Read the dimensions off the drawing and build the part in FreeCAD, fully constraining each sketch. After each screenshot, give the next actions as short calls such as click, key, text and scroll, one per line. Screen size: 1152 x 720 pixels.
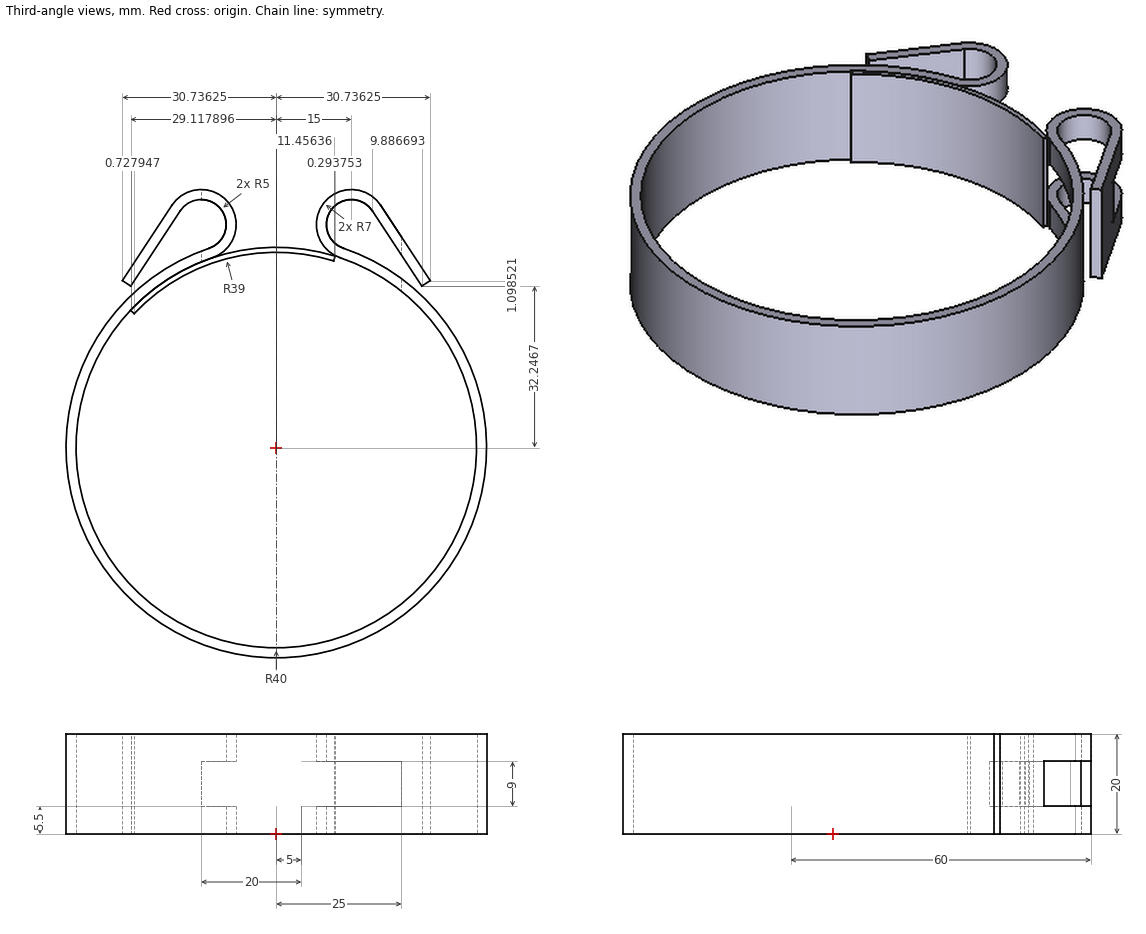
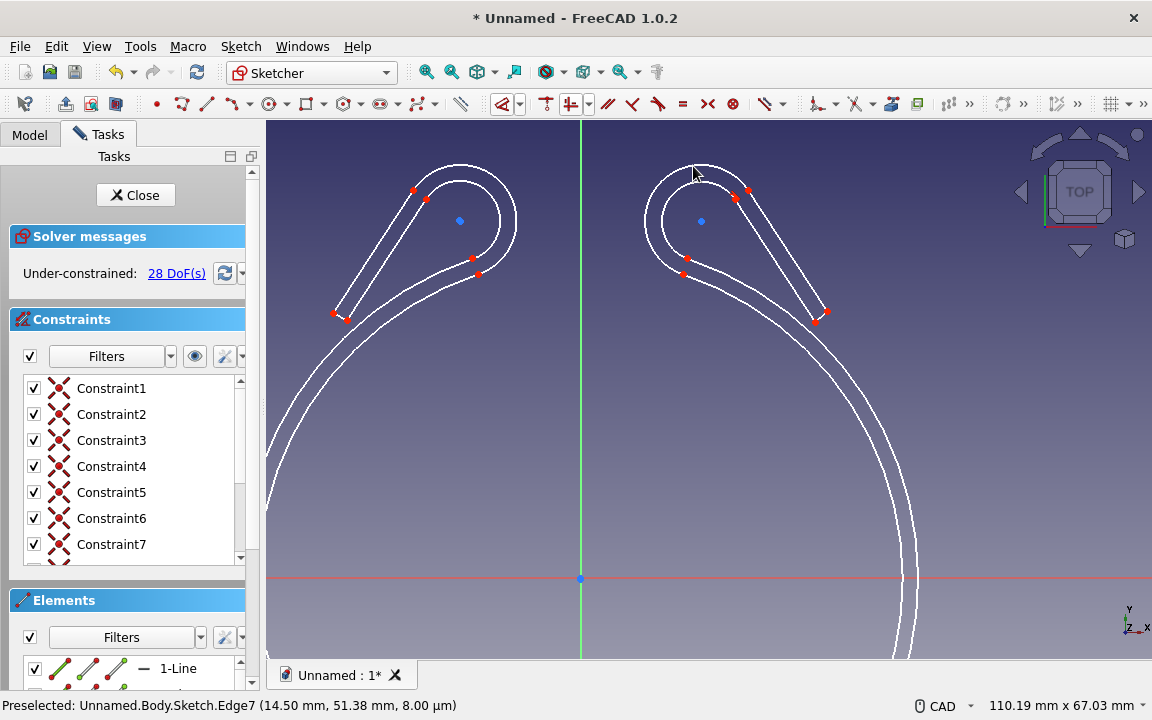
click(389, 227)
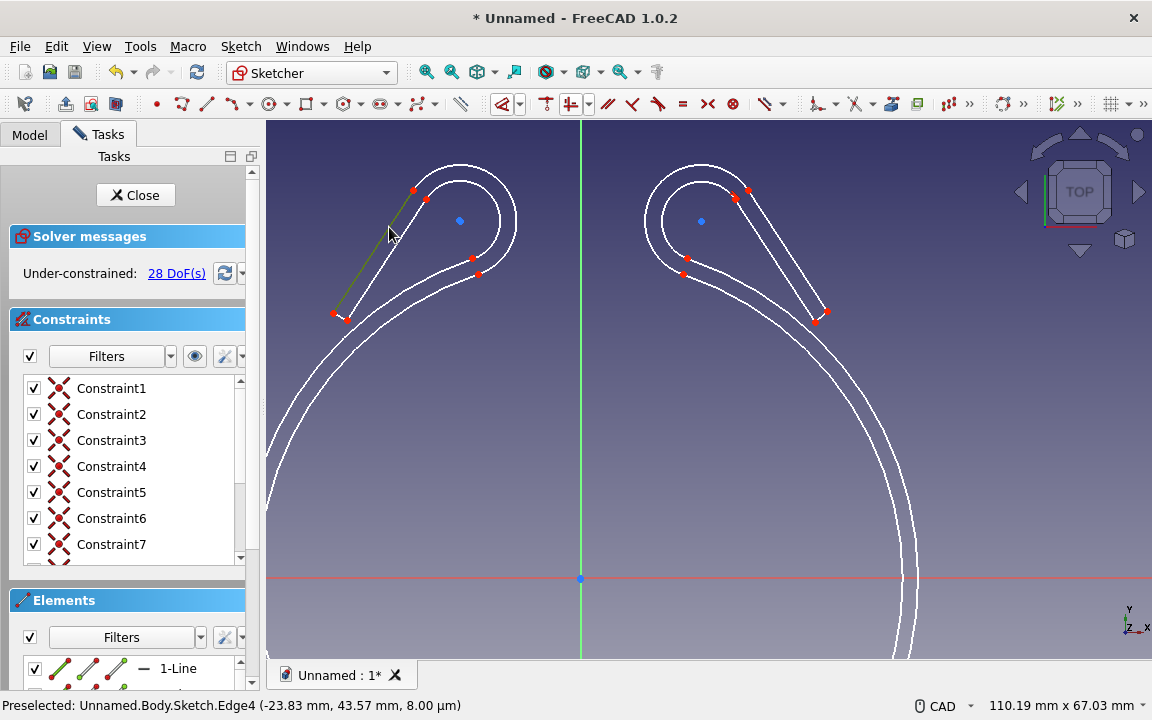
click(516, 227)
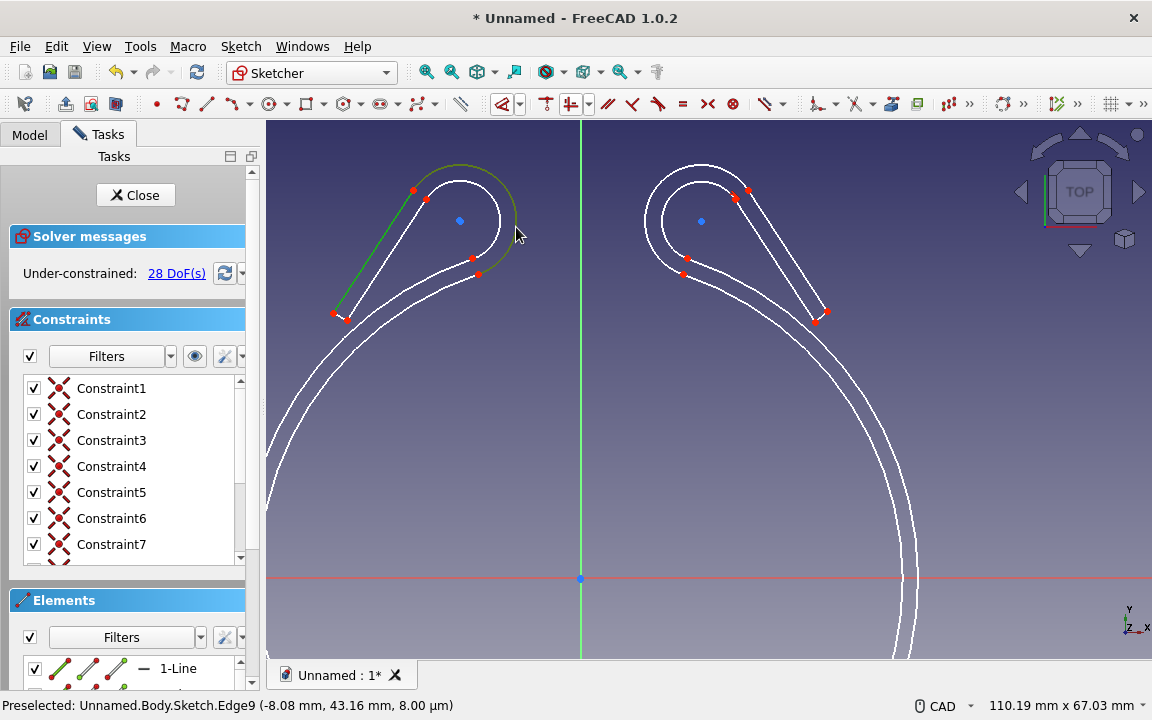
key(t)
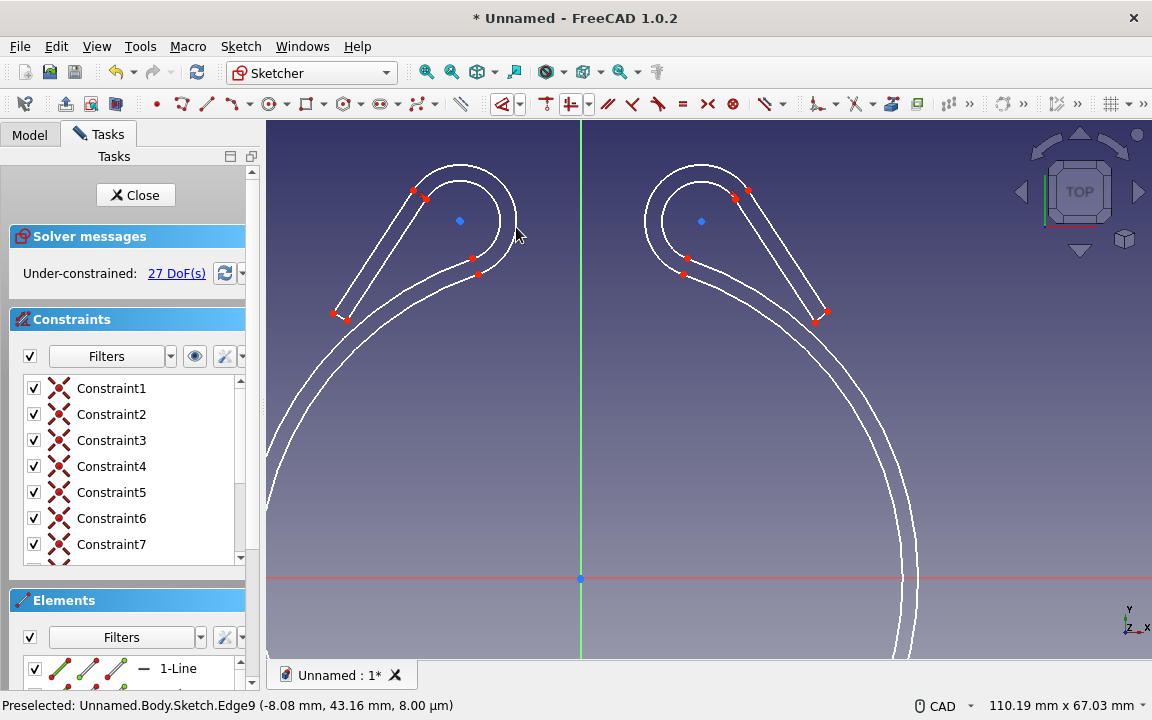
click(371, 284)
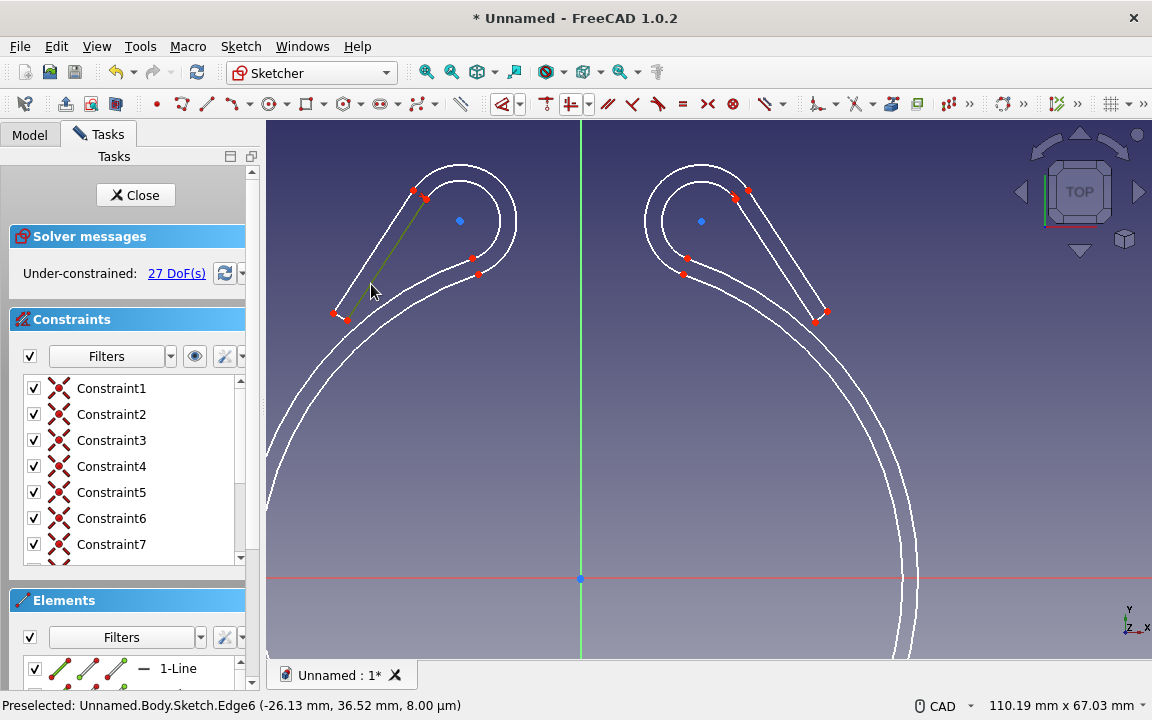
click(500, 225)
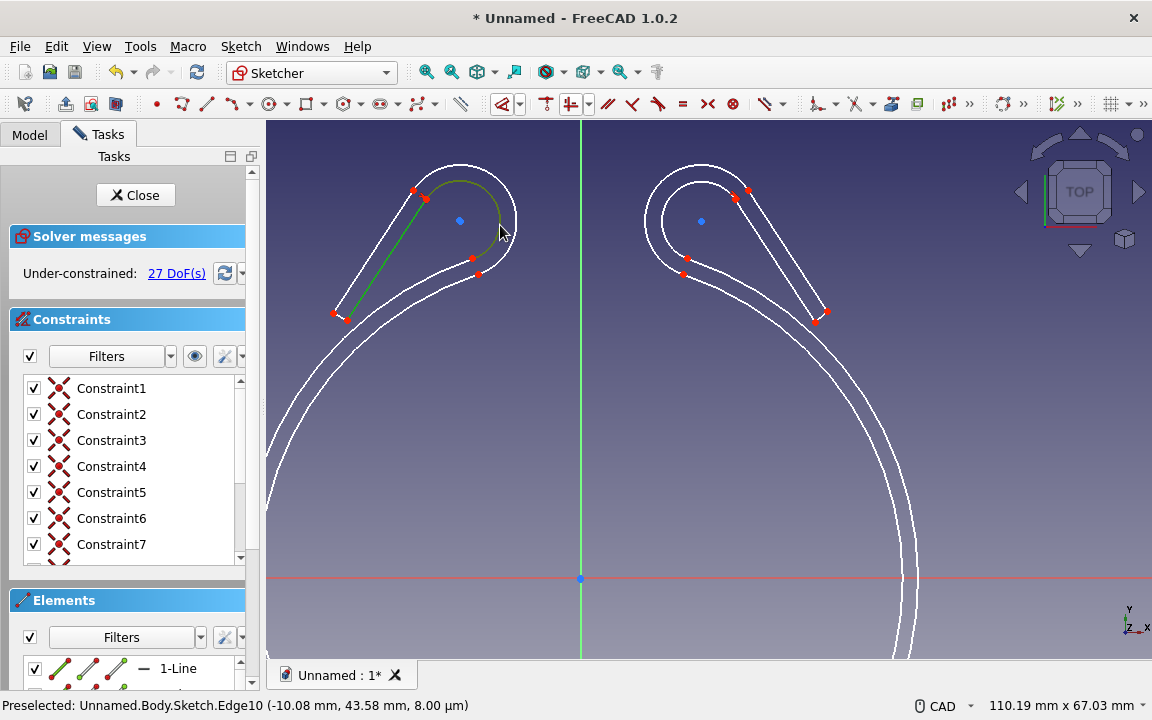
click(658, 104)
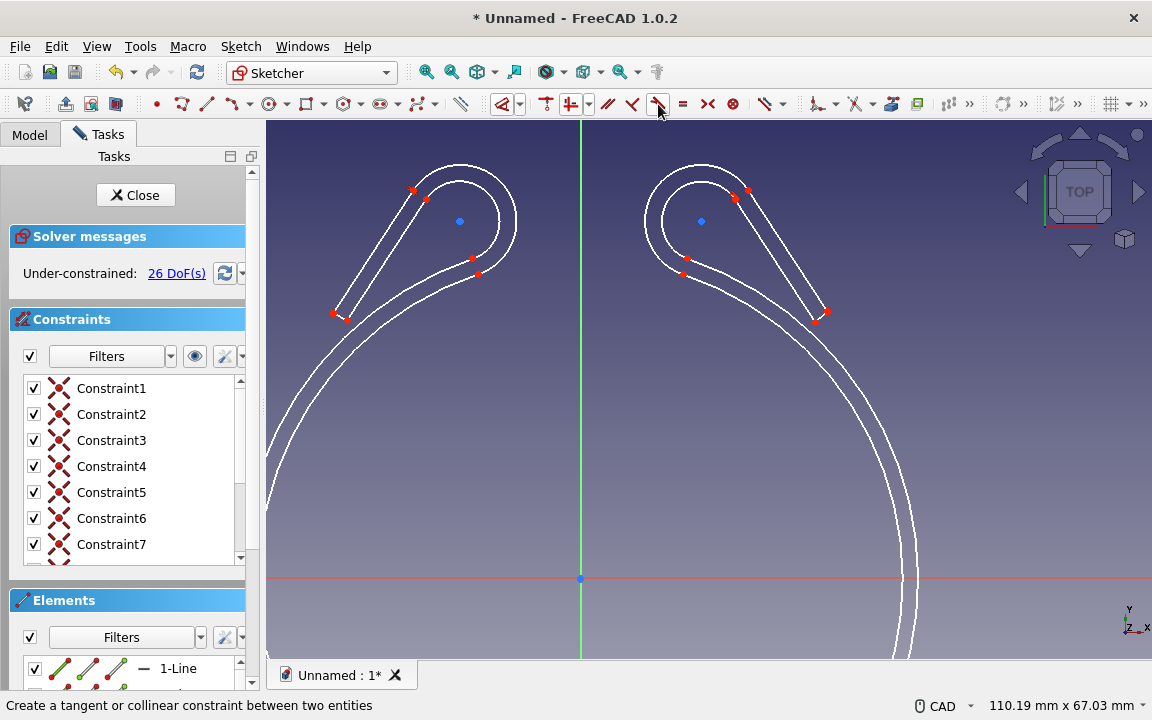
click(693, 166)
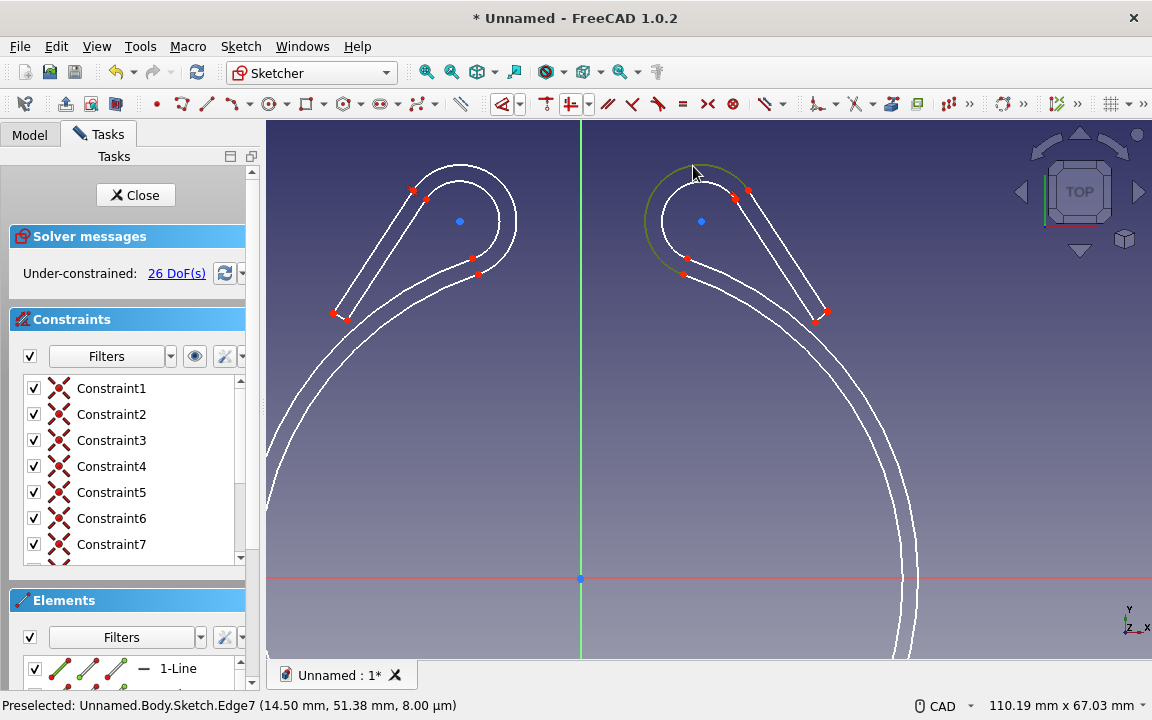
click(900, 541)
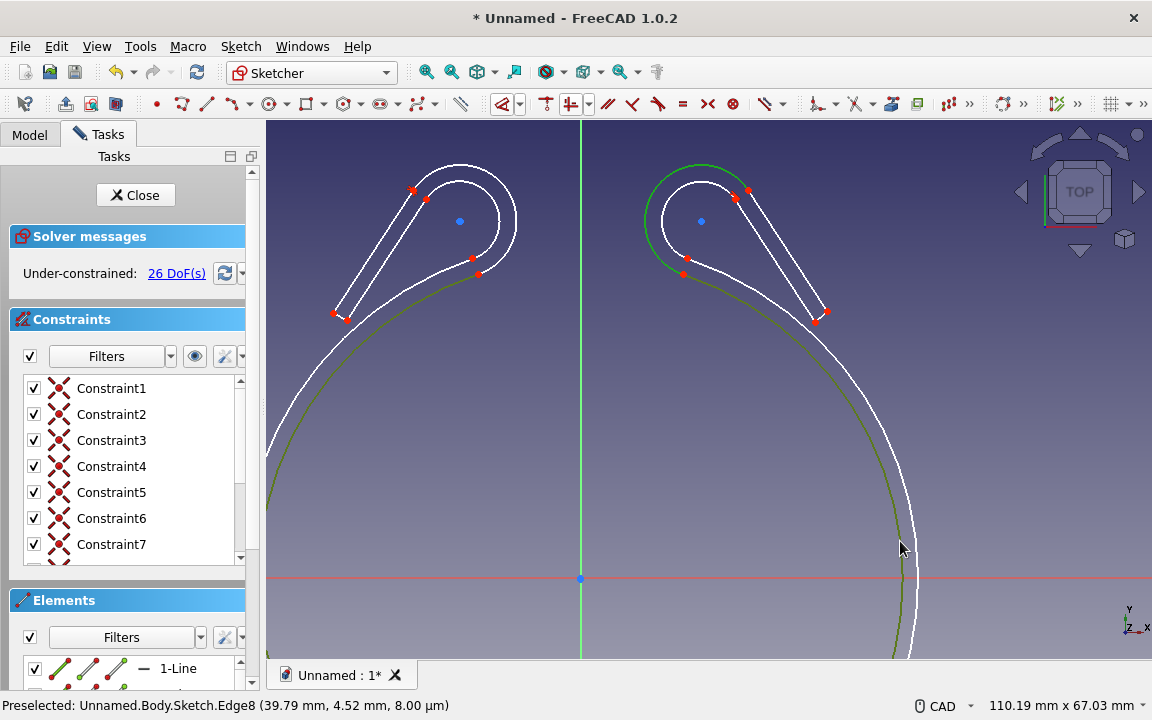
key(t)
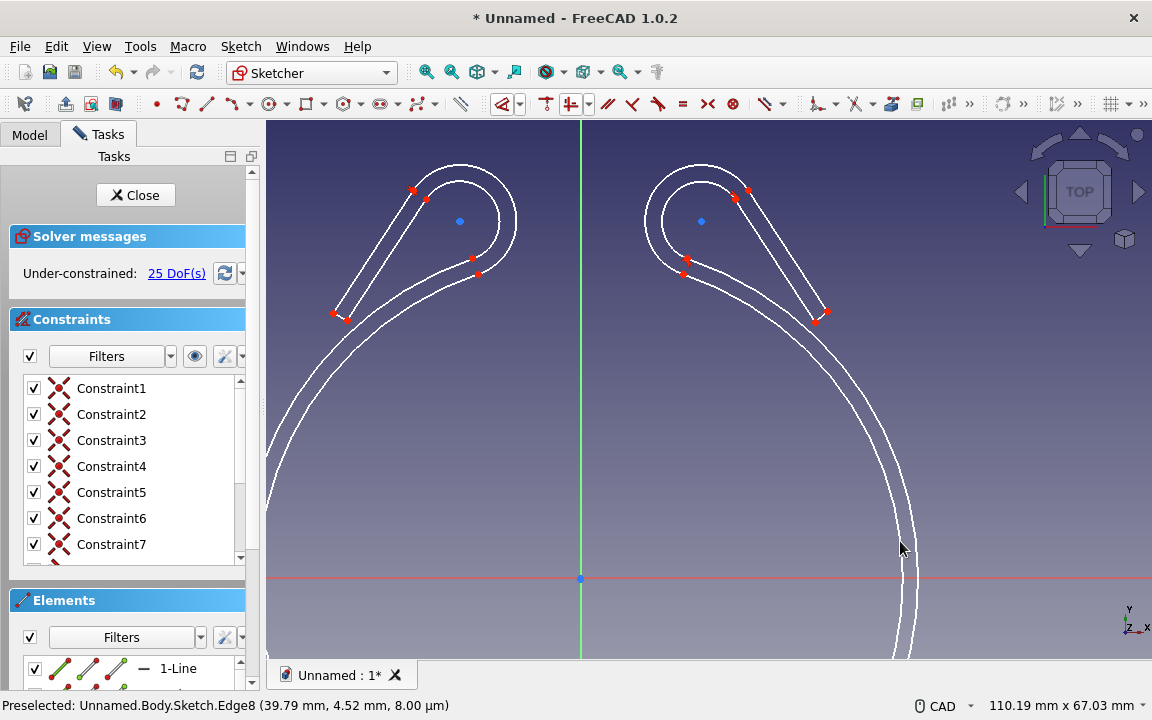
click(901, 542)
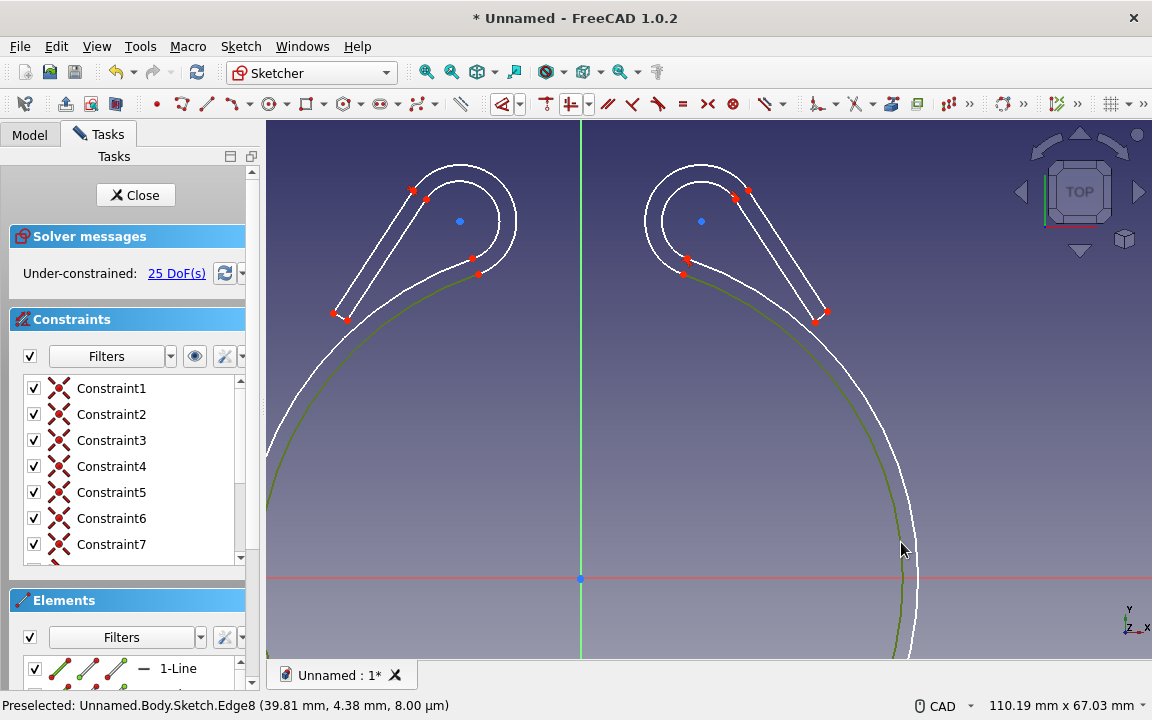
click(516, 227)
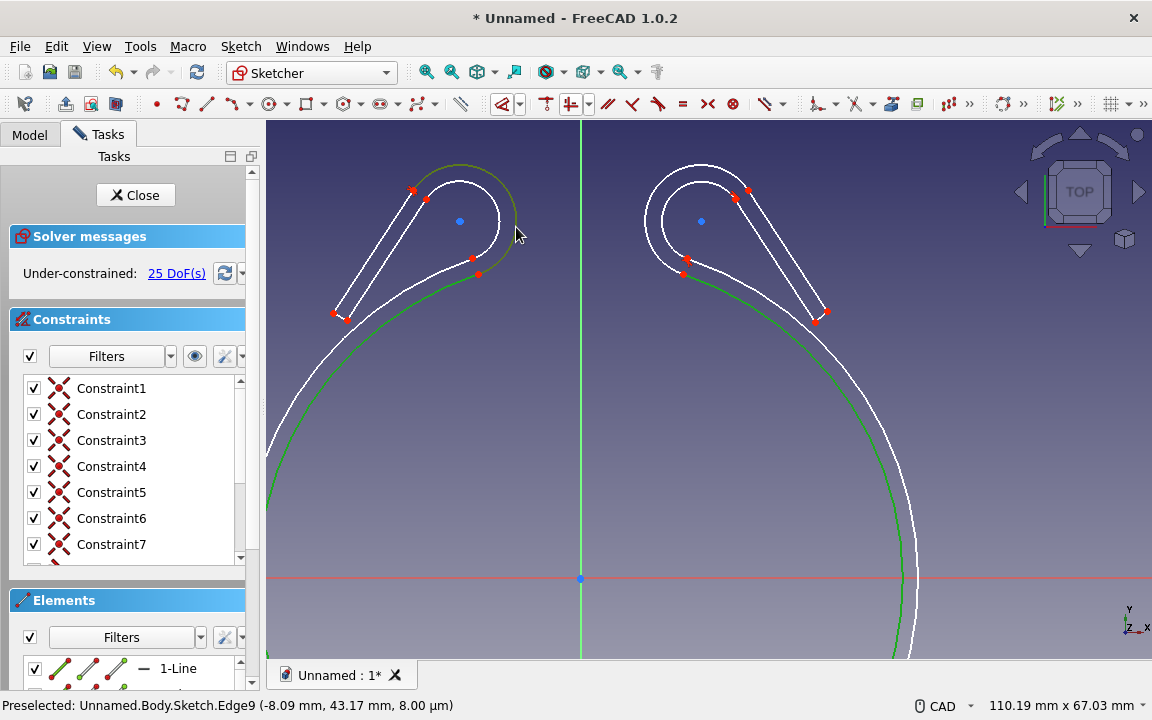
click(658, 104)